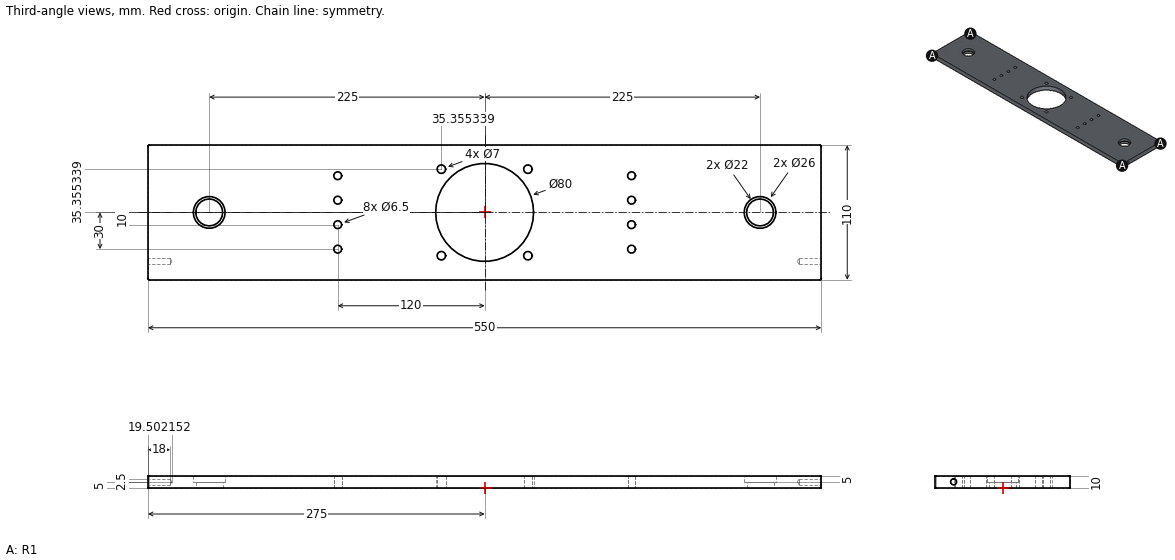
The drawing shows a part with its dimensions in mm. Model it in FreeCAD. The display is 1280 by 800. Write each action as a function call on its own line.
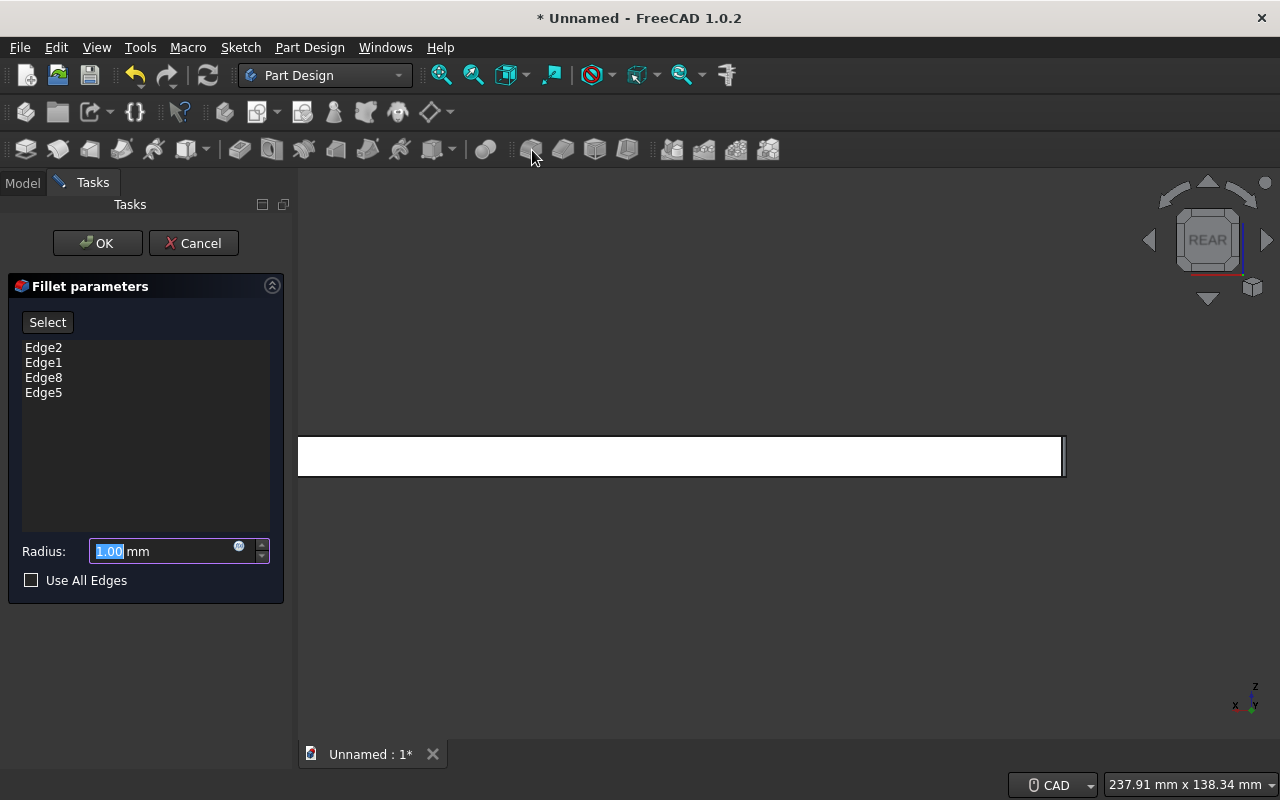
text(1)
key(Tab)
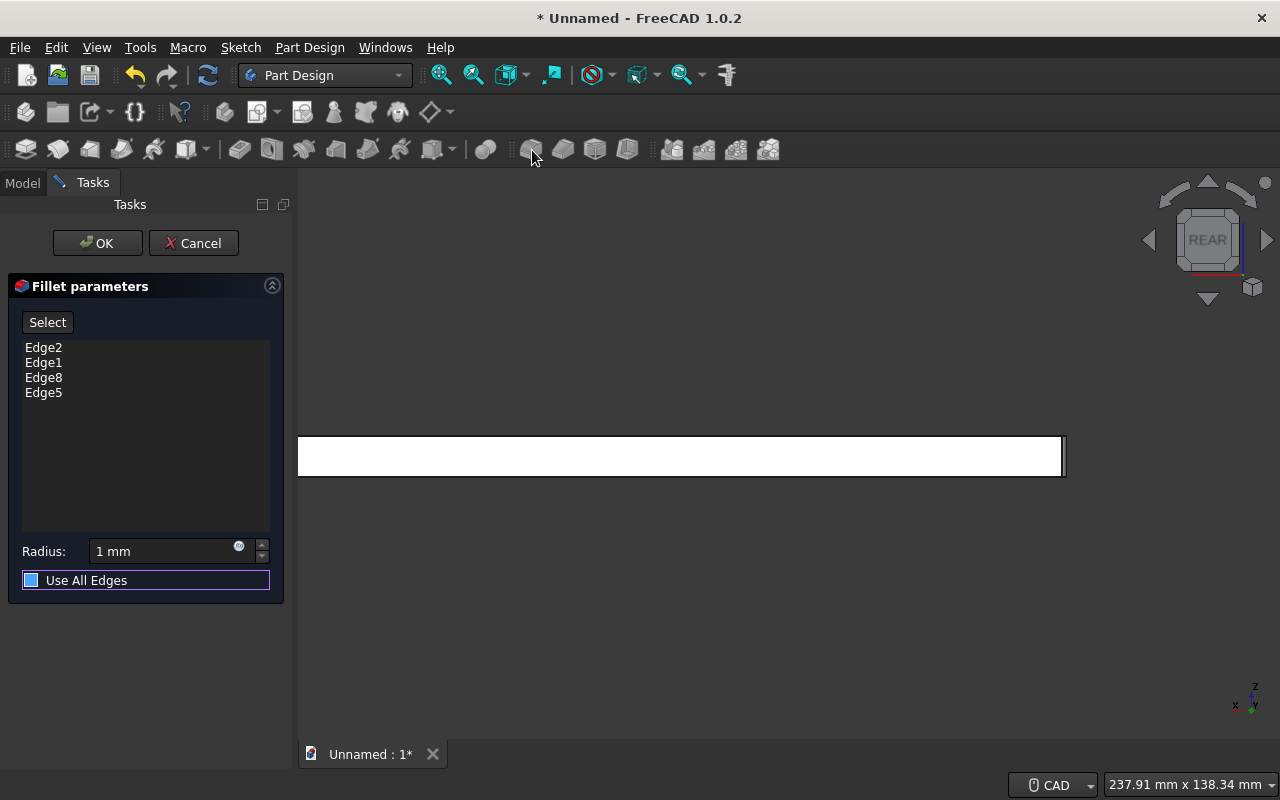
click(98, 243)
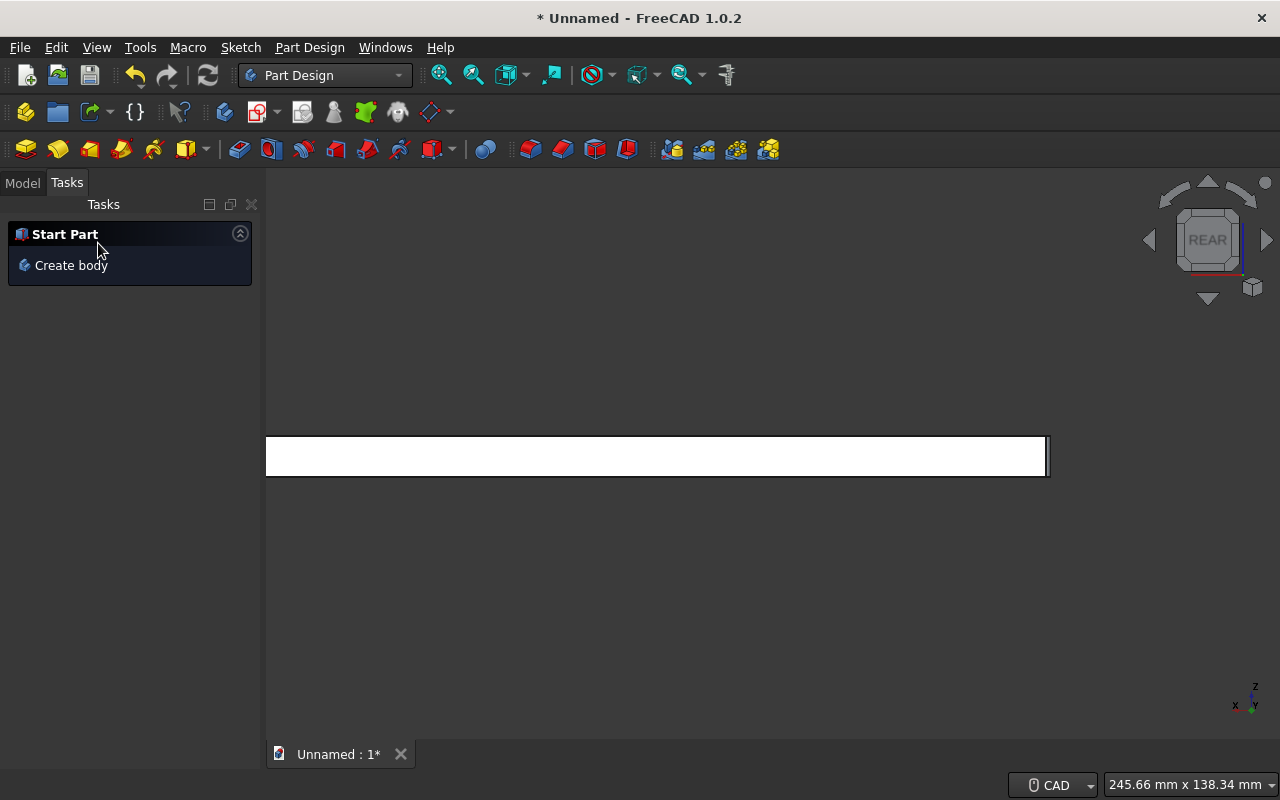
key(v)
key(f)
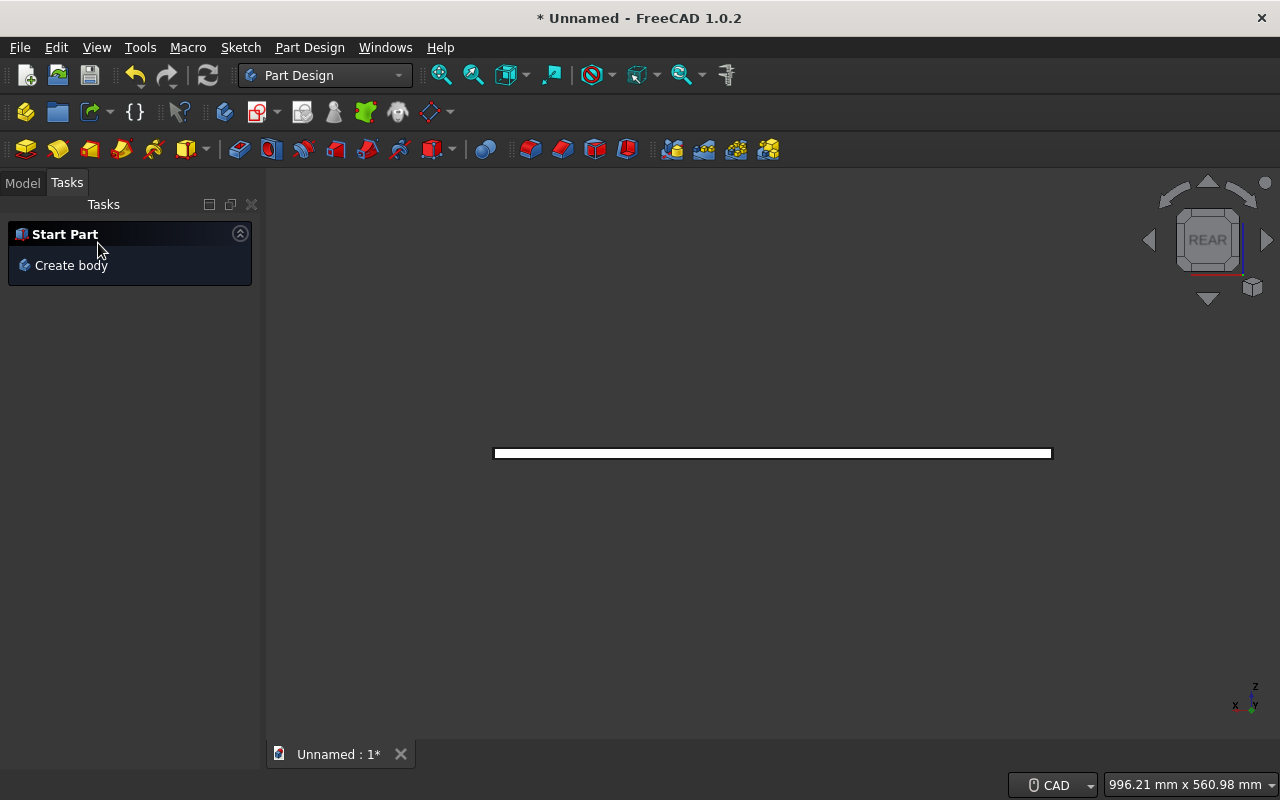
click(23, 182)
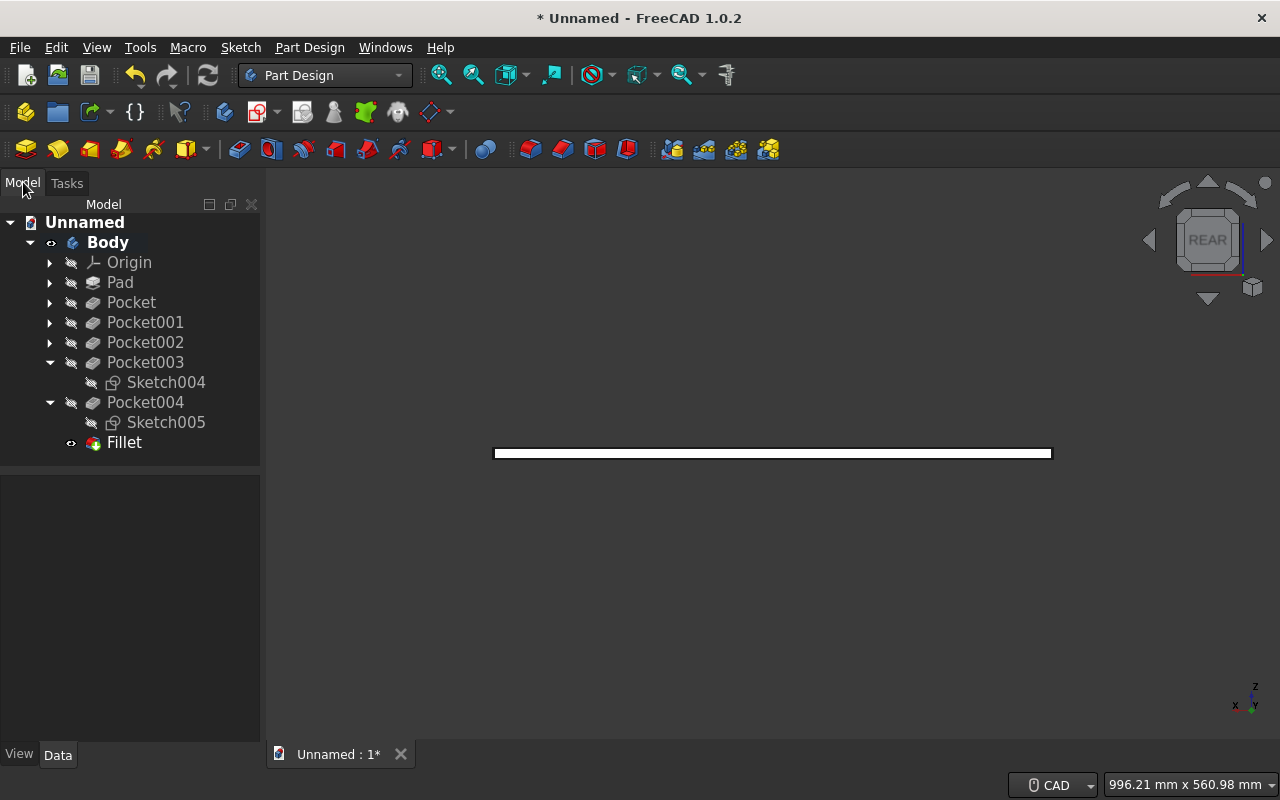
click(50, 263)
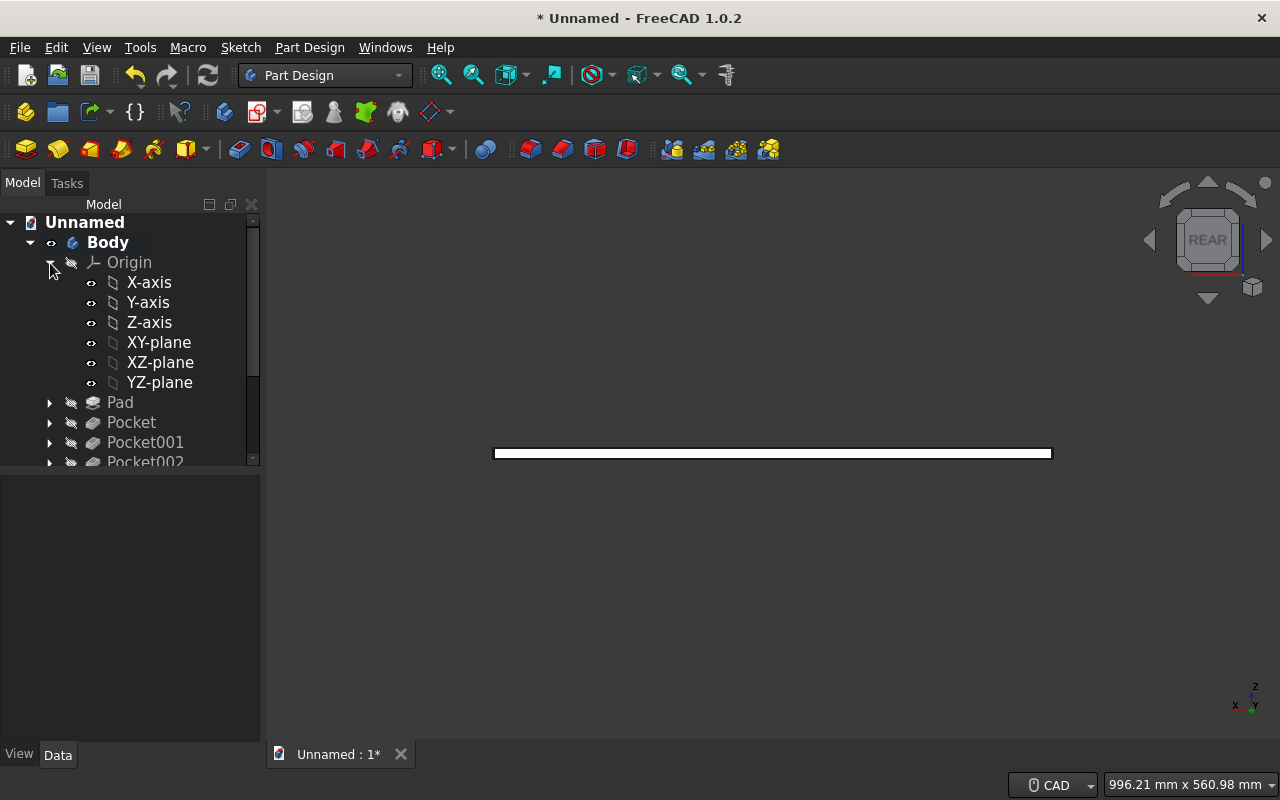
click(136, 363)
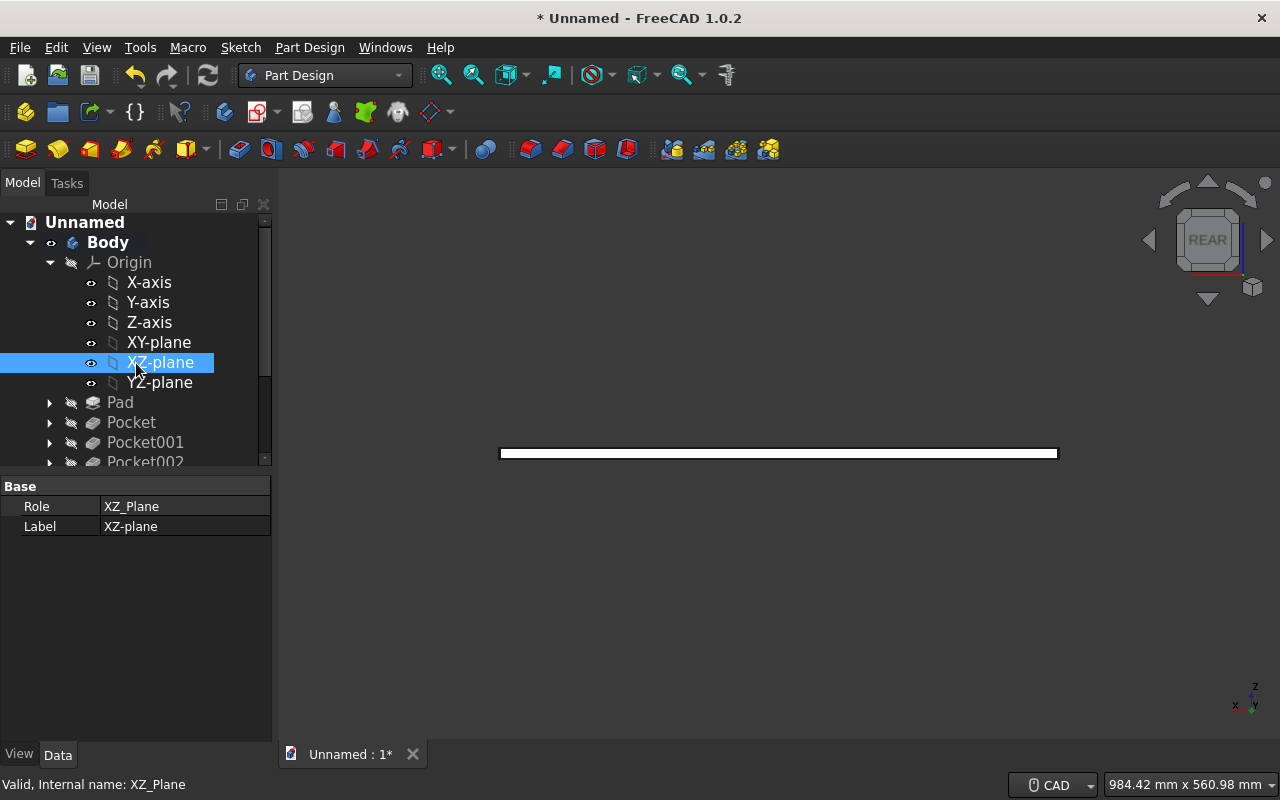
click(430, 112)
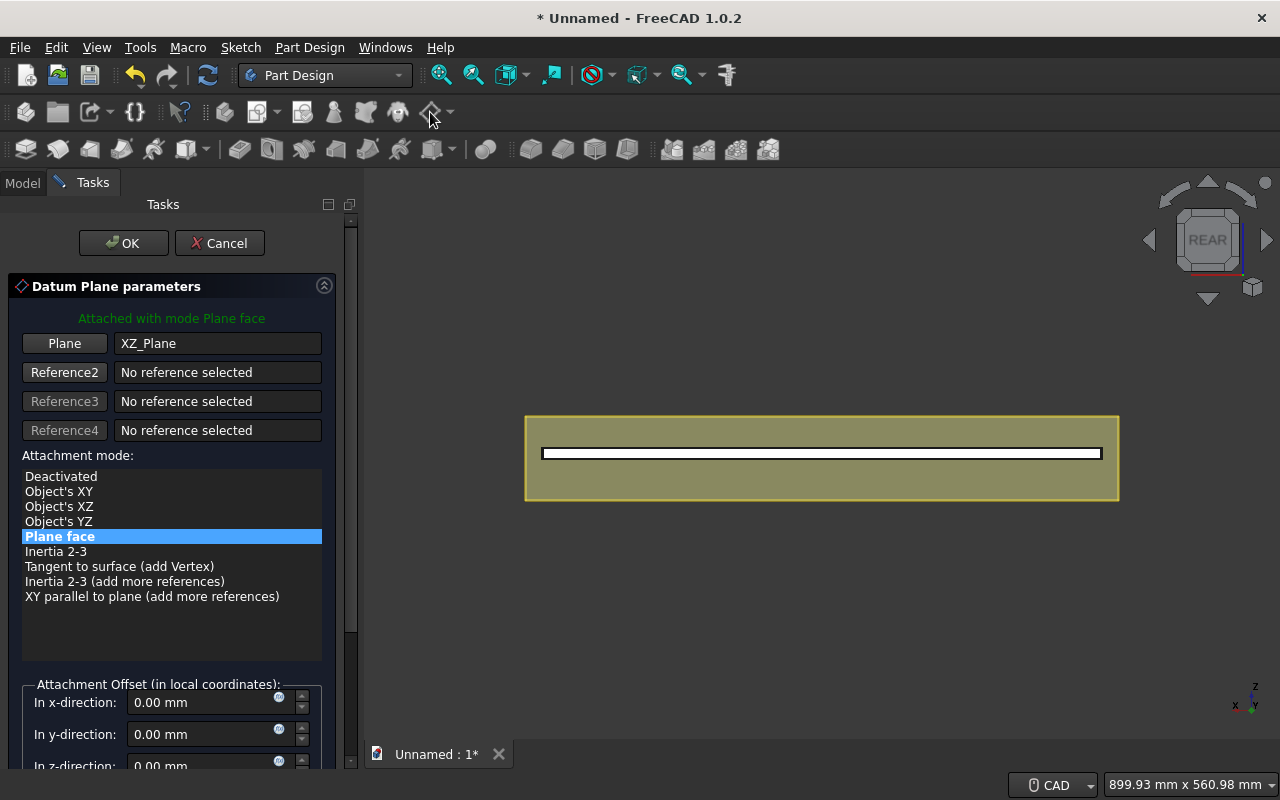
scroll(351, 491, down, 2)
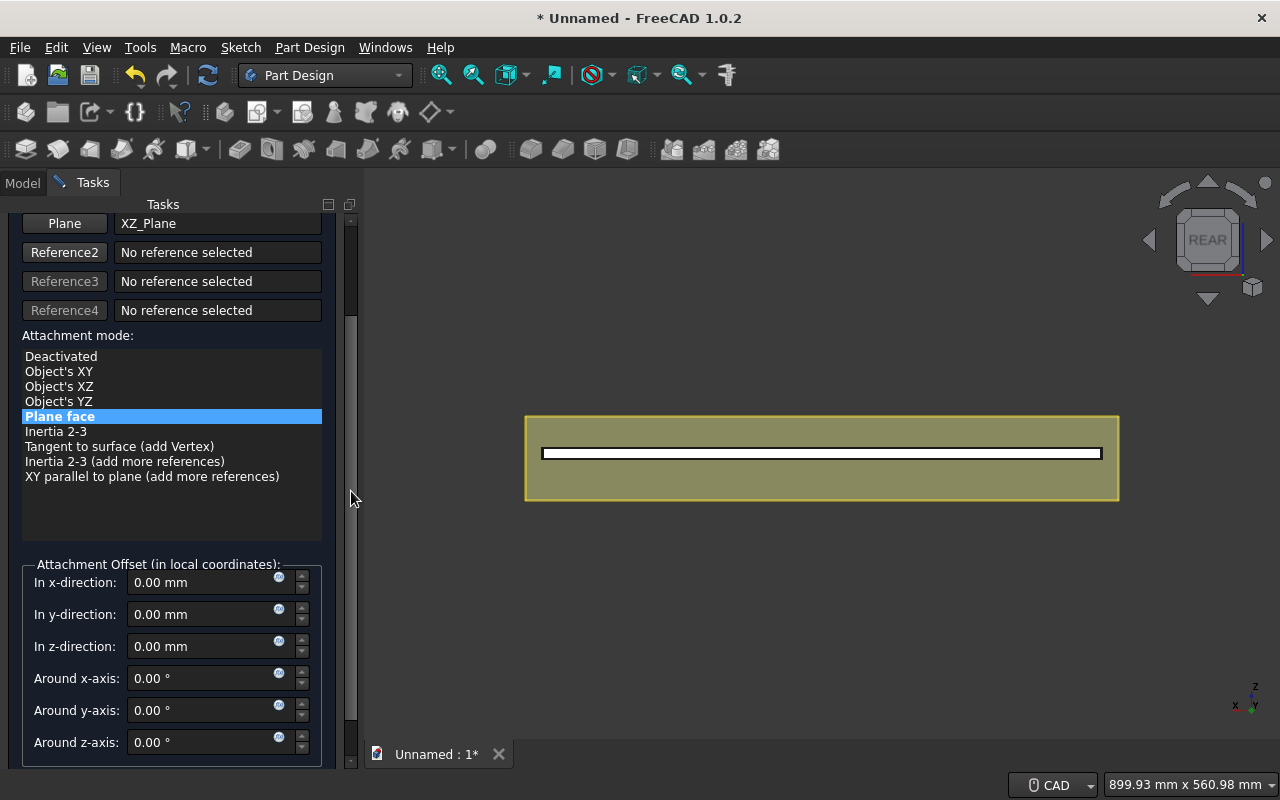
triple_click(210, 646)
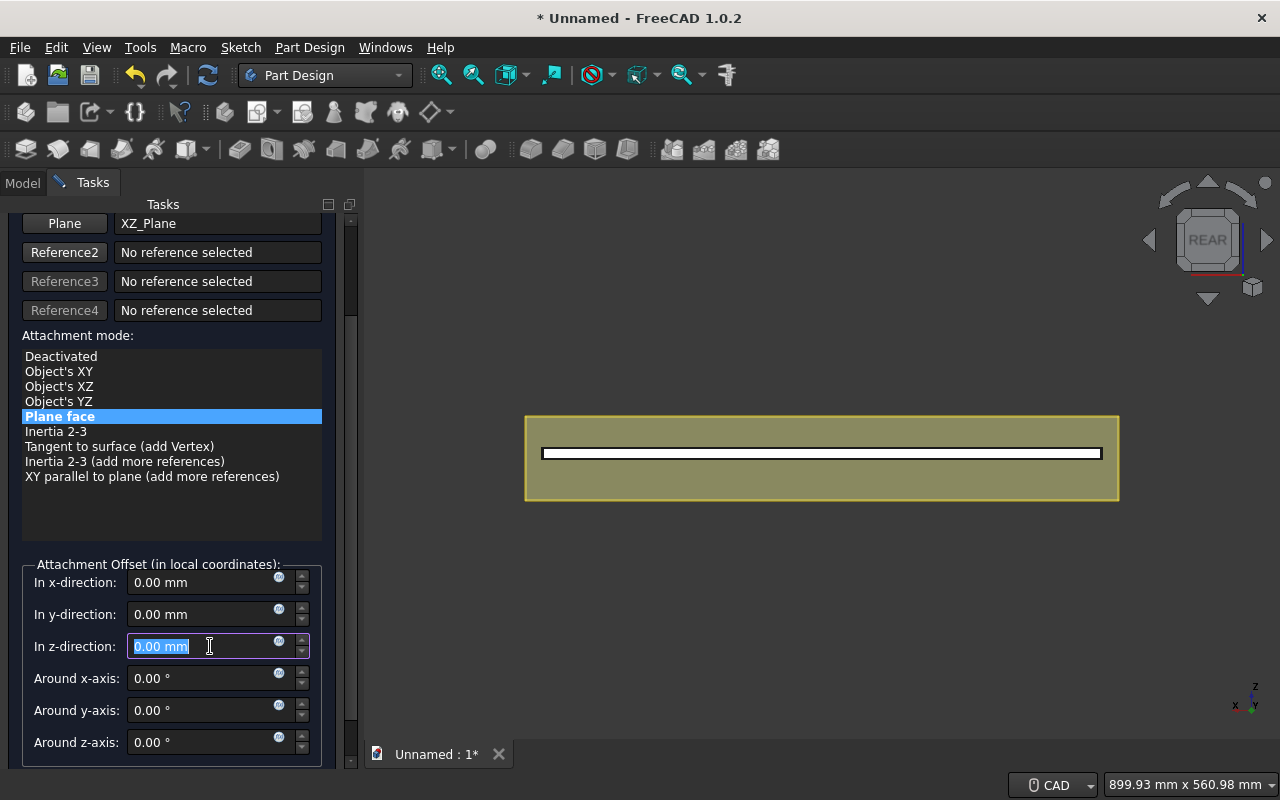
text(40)
key(Tab)